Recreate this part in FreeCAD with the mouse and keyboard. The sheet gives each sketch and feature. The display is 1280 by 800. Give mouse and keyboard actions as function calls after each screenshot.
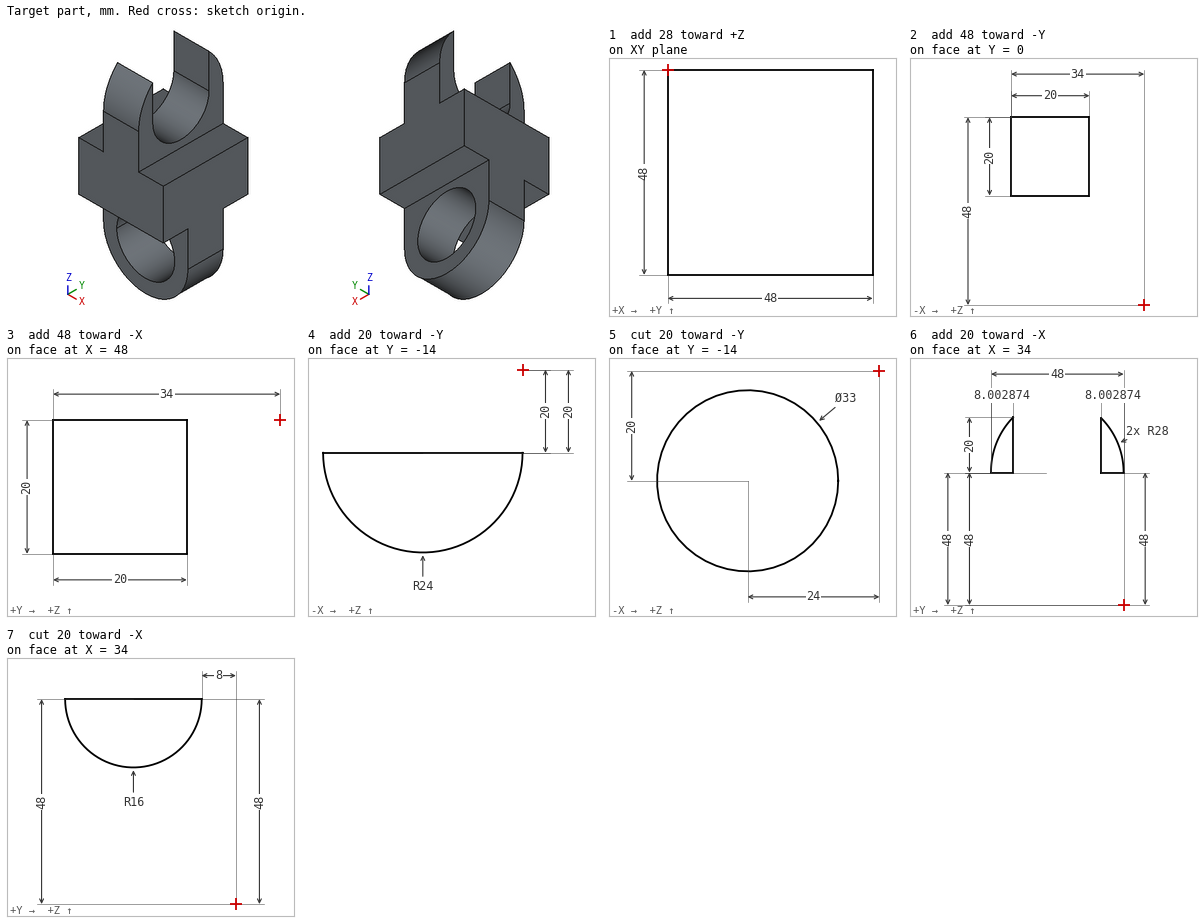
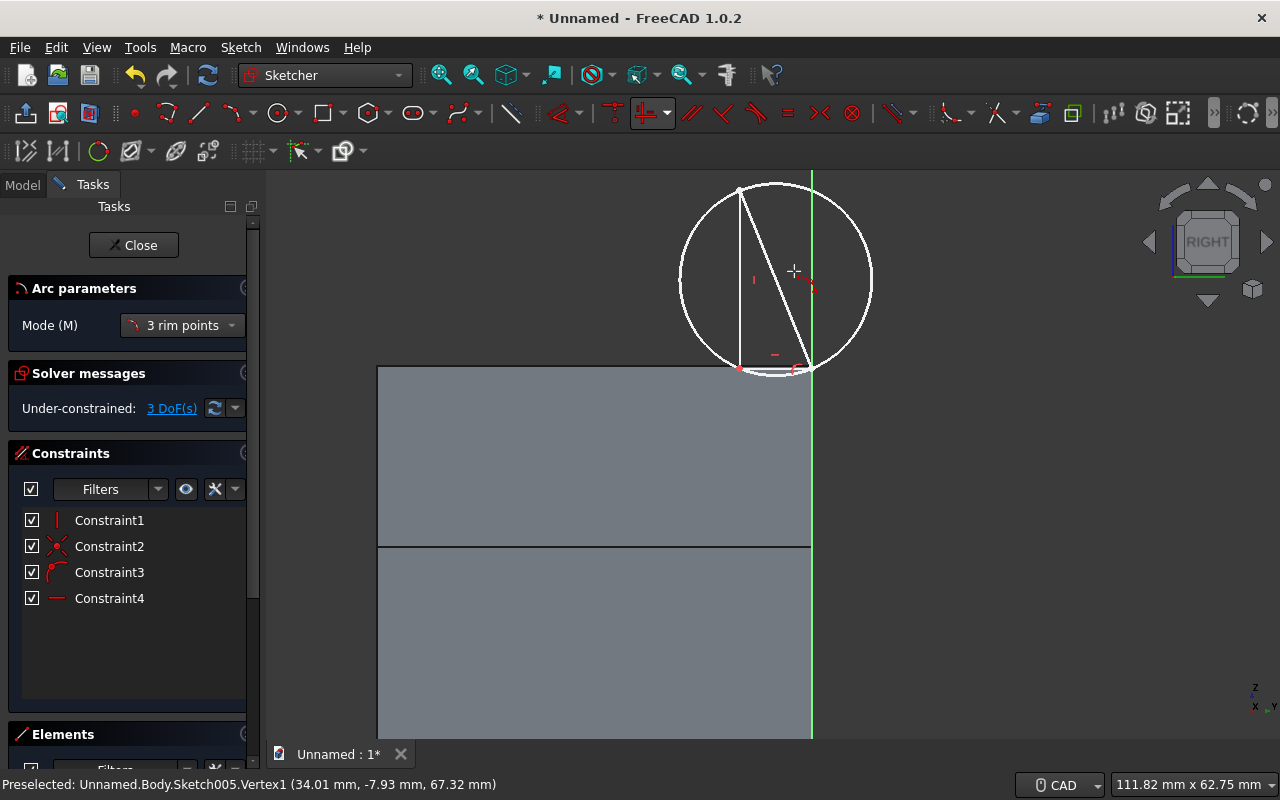
click(793, 270)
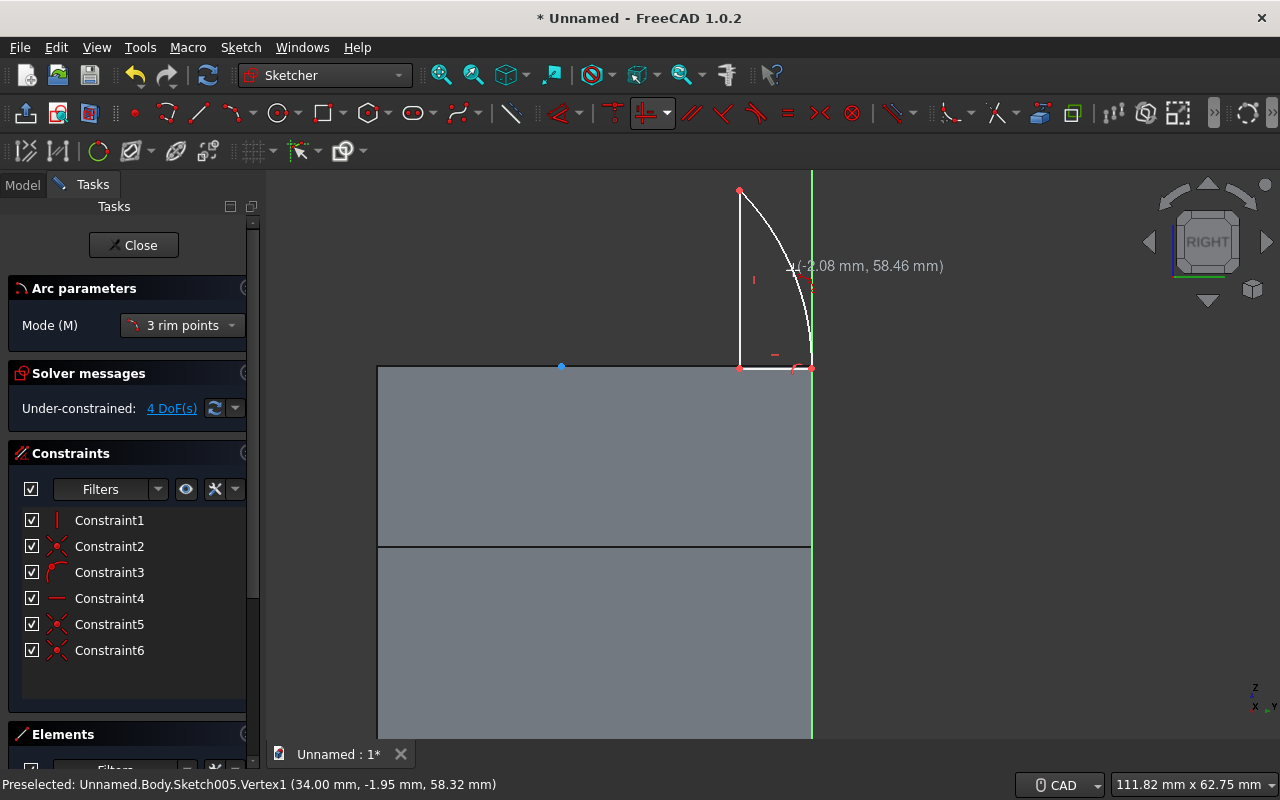
key(g)
key(m)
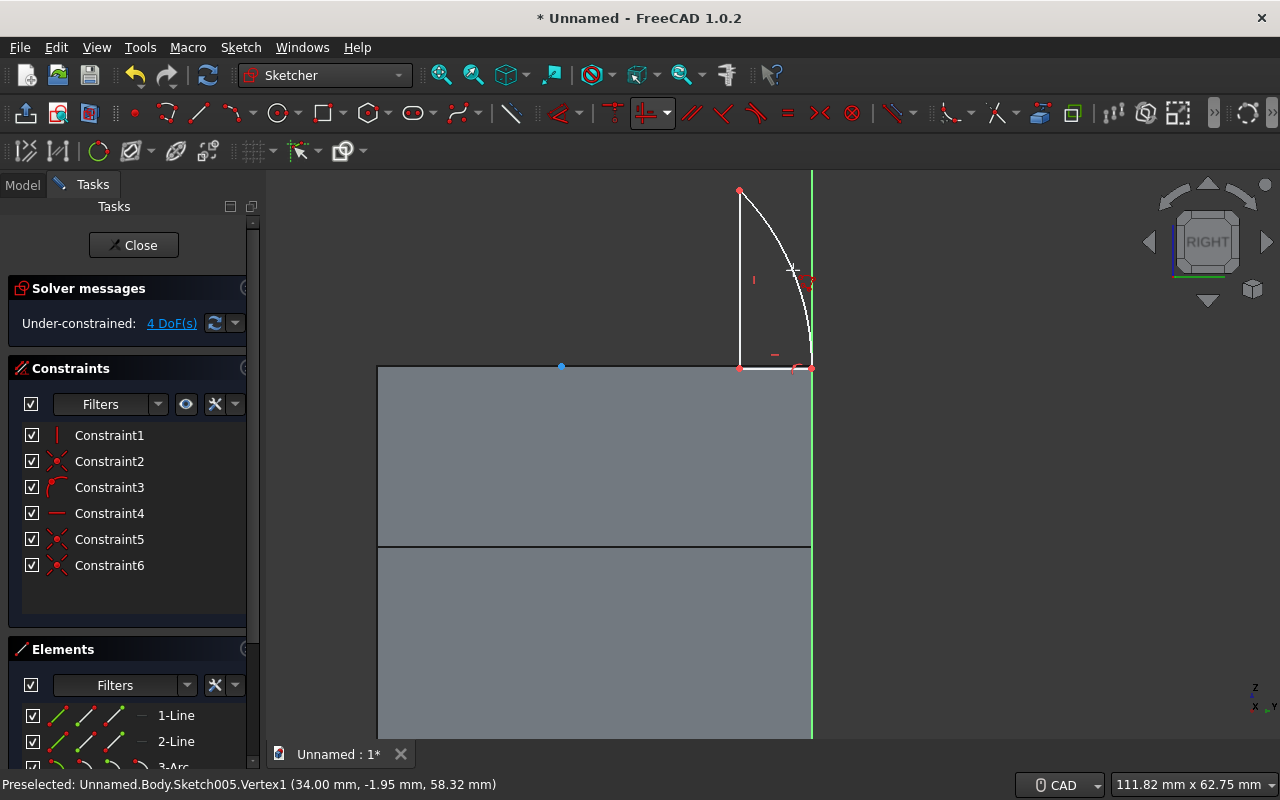
click(377, 366)
click(449, 366)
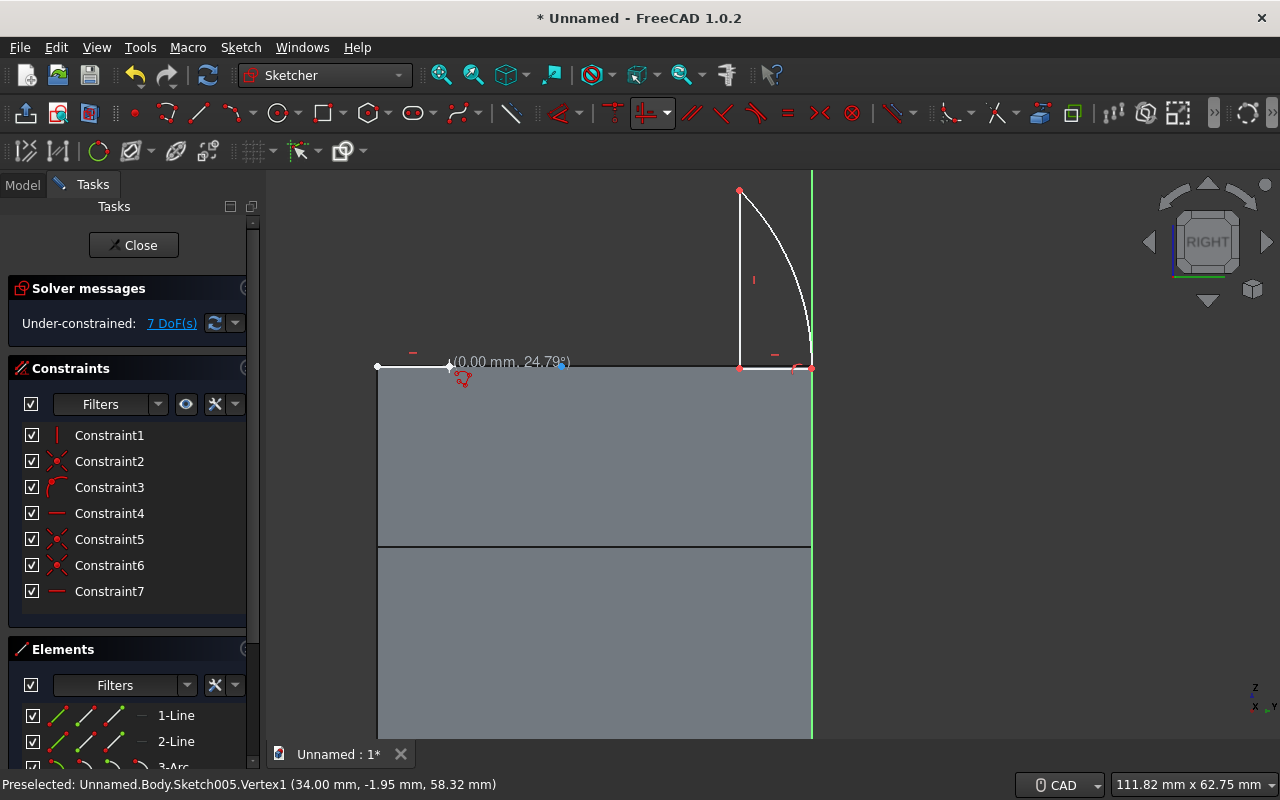
scroll(839, 408, down, 3)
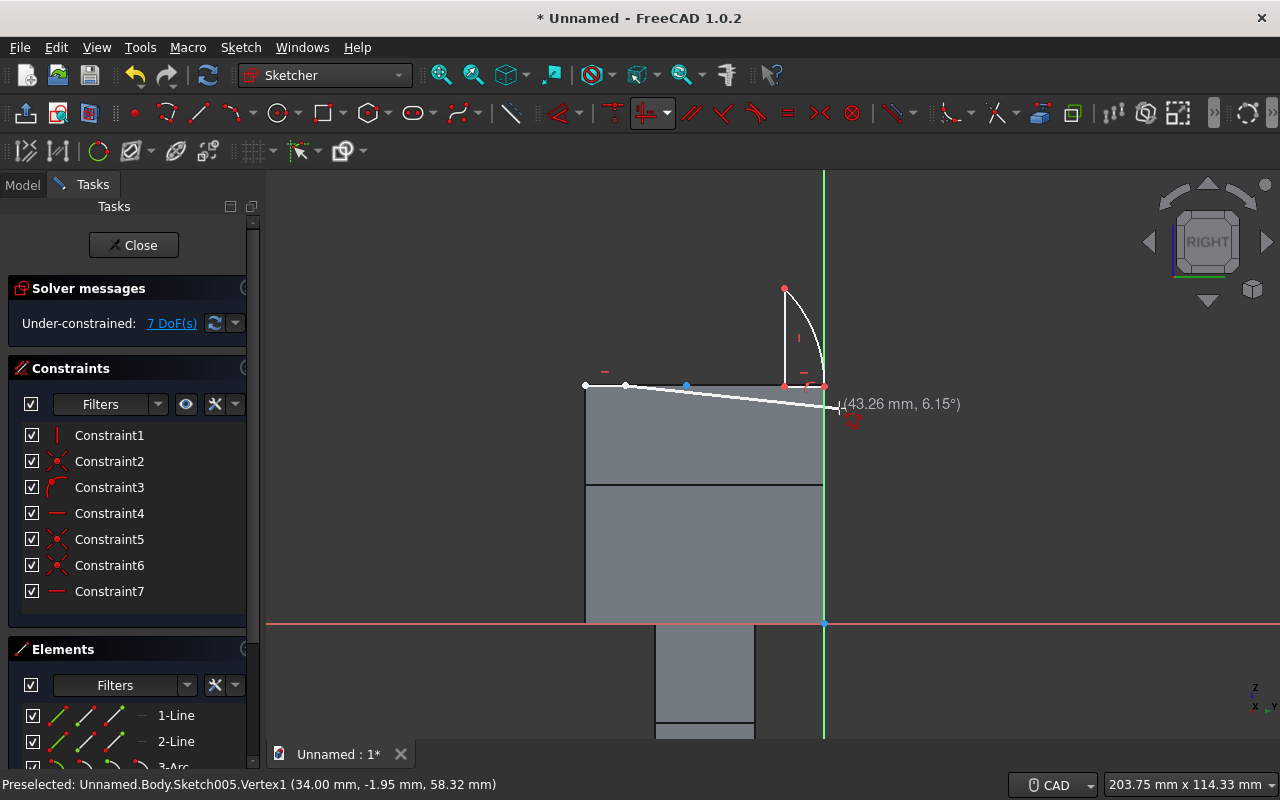
click(625, 286)
right_click(625, 286)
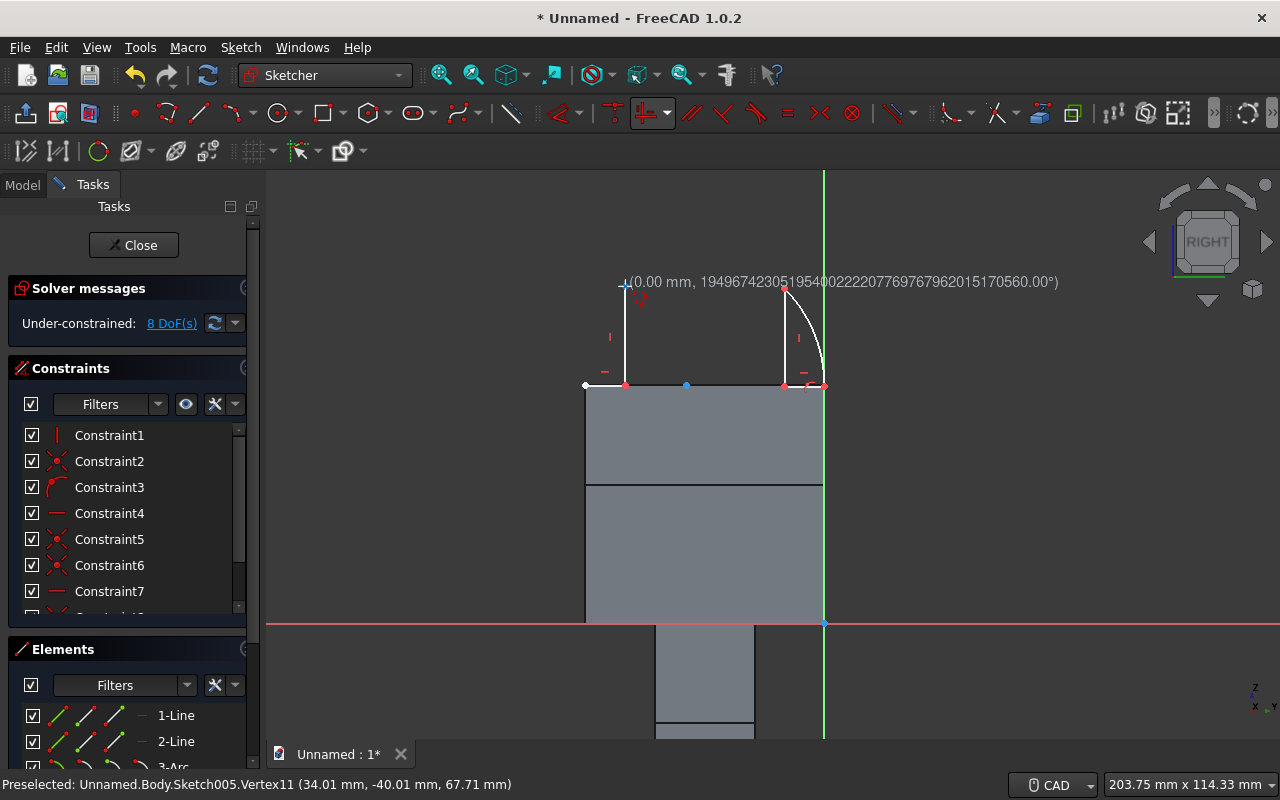
click(232, 114)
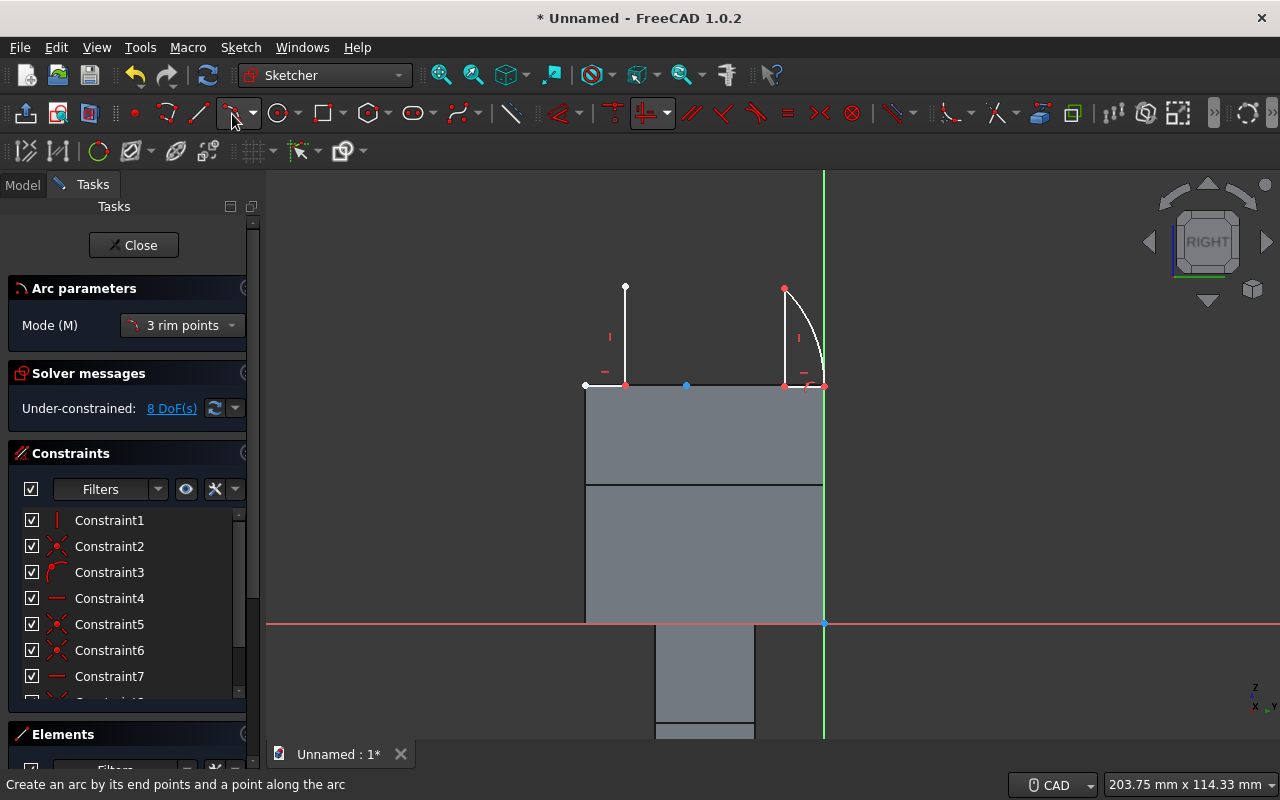
click(625, 287)
click(586, 386)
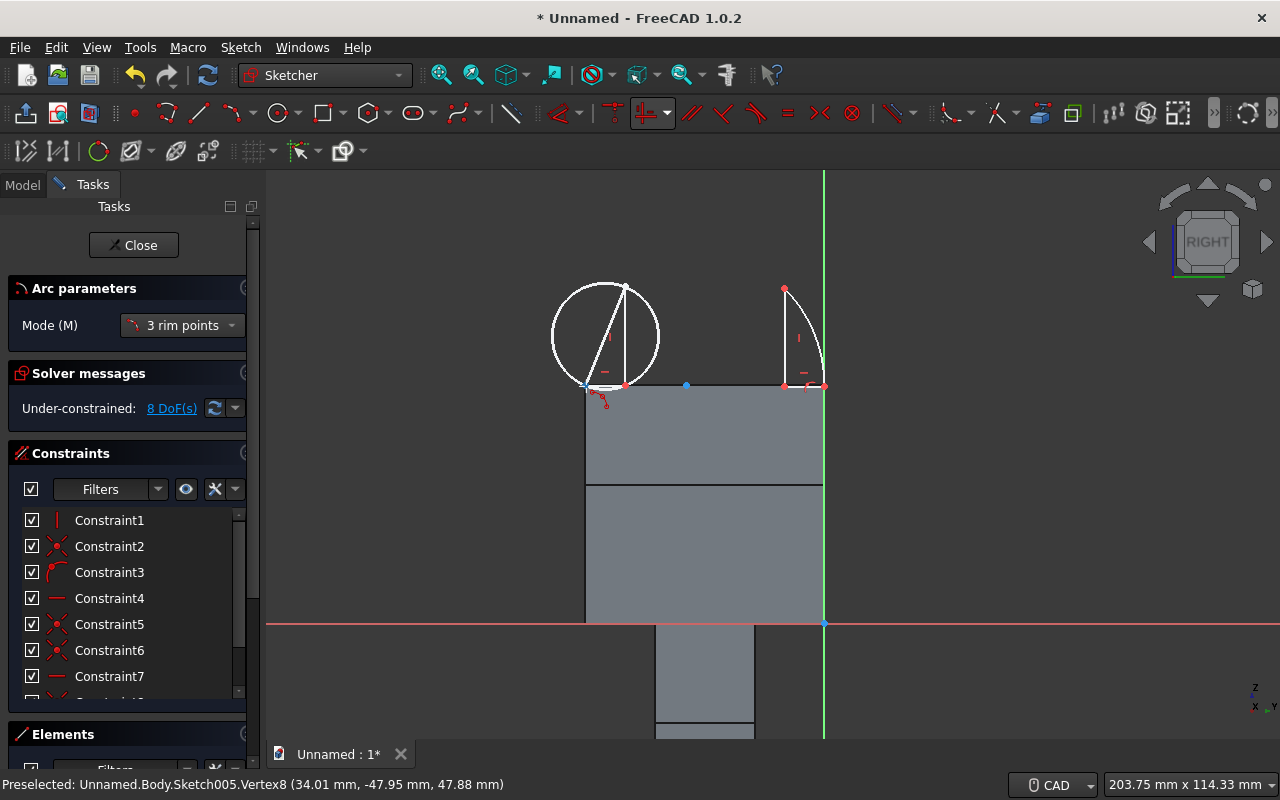
scroll(595, 331, up, 2)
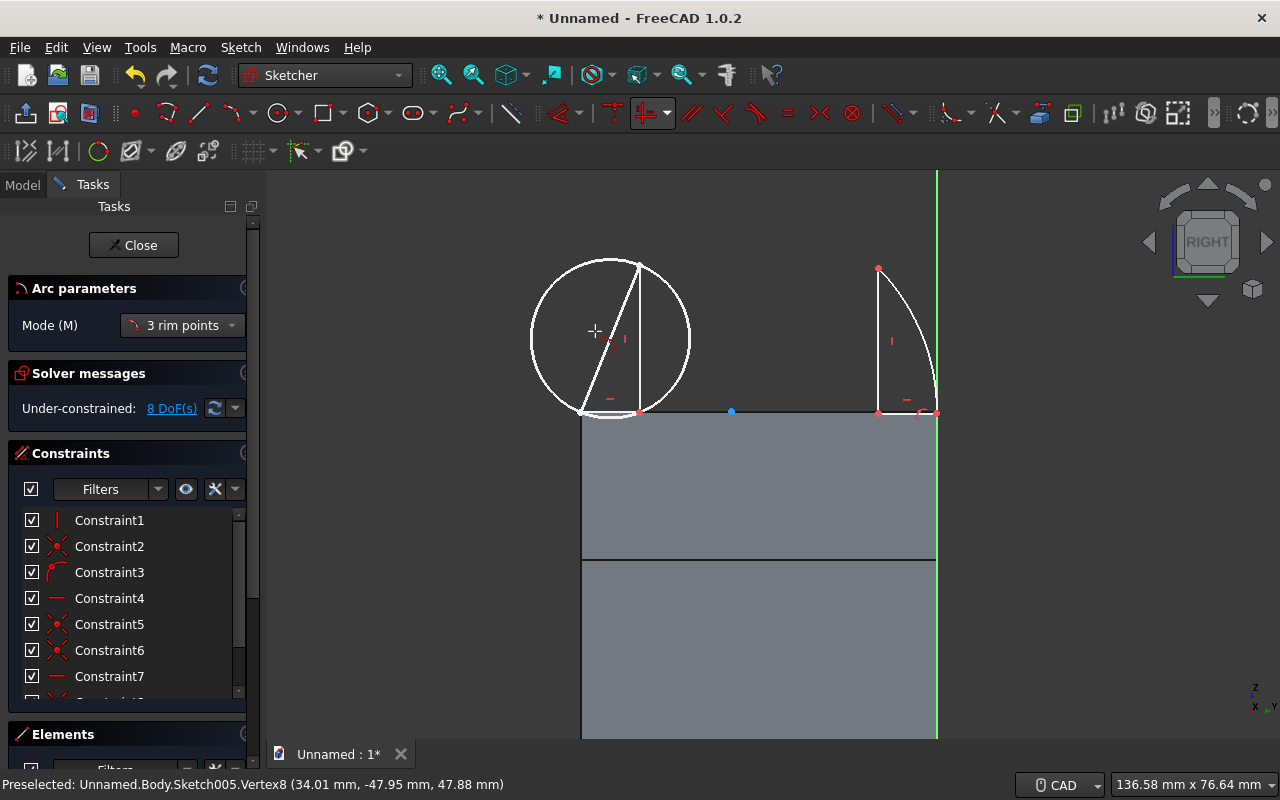
click(595, 331)
key(Escape)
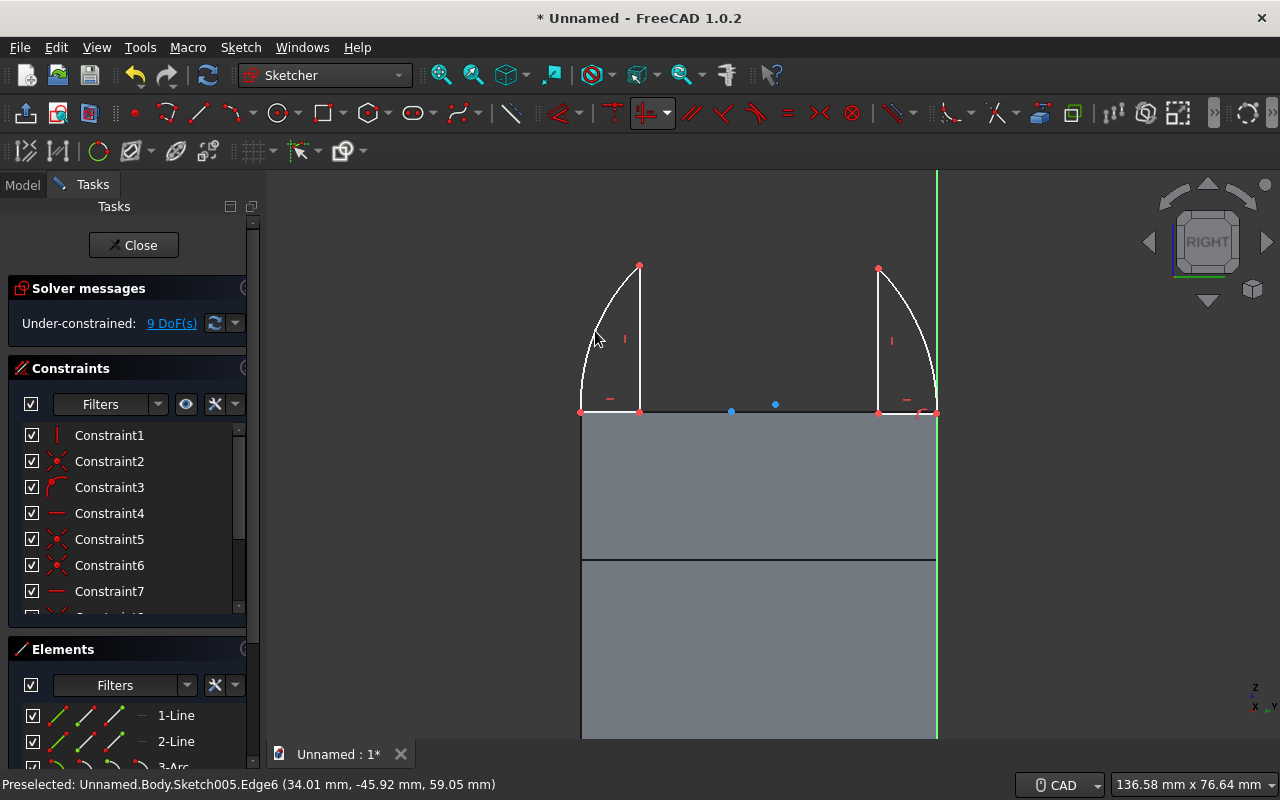
click(908, 306)